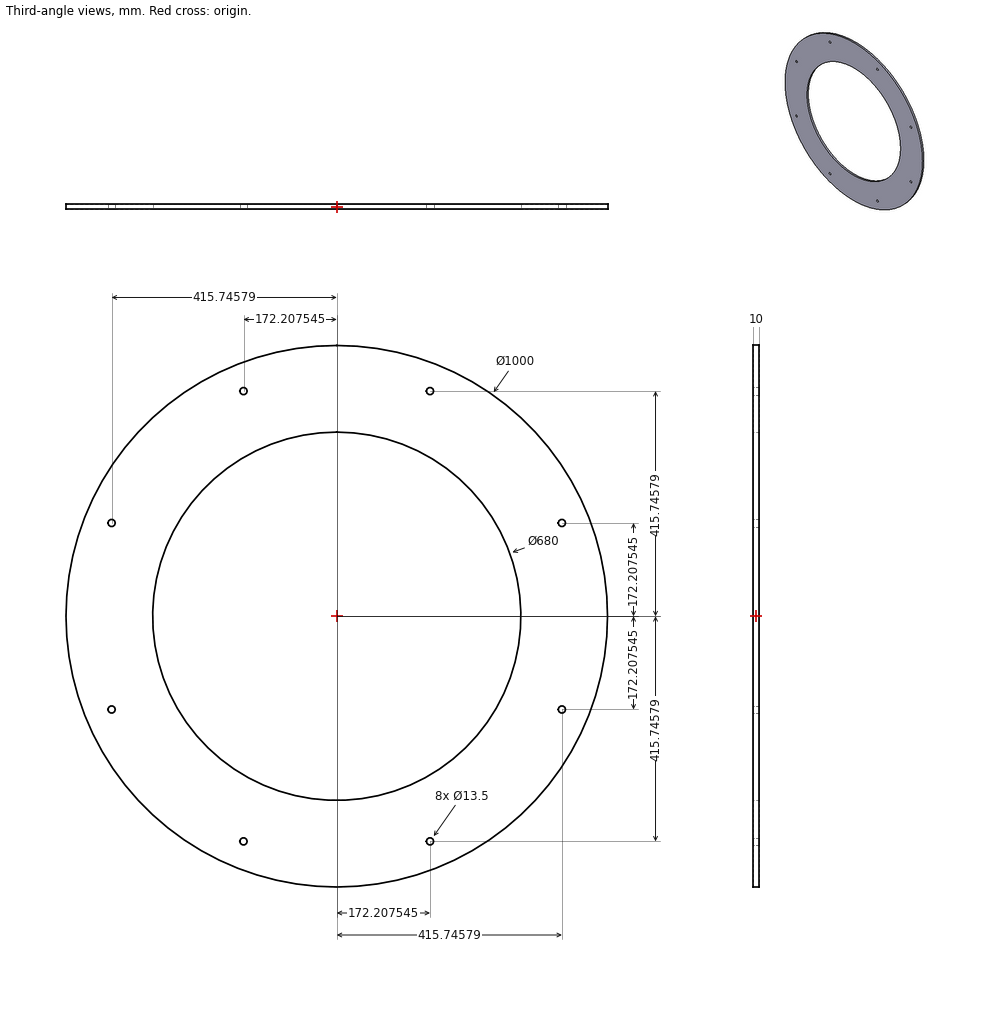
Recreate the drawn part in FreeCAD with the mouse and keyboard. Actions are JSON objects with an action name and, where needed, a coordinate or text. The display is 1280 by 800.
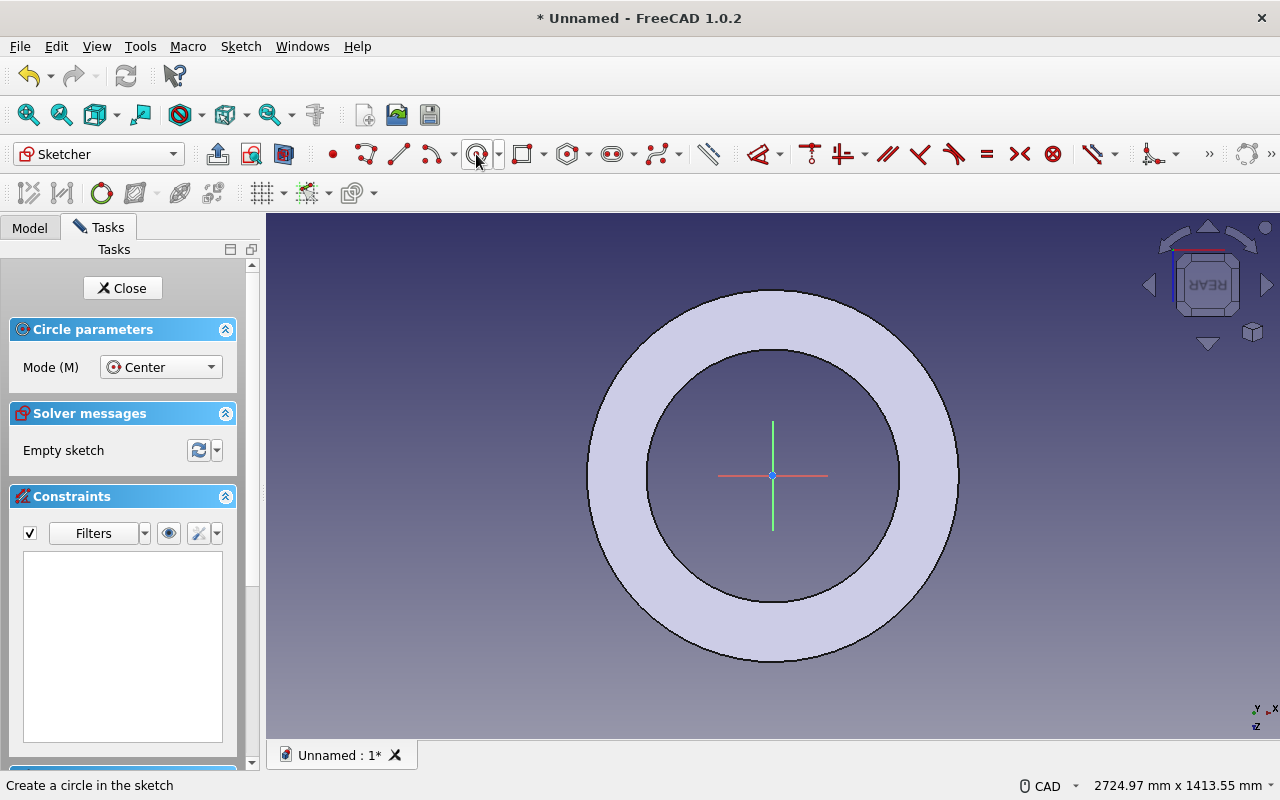
{"action": "scroll", "coordinate": [837, 321], "scroll_direction": "up", "scroll_amount": 12}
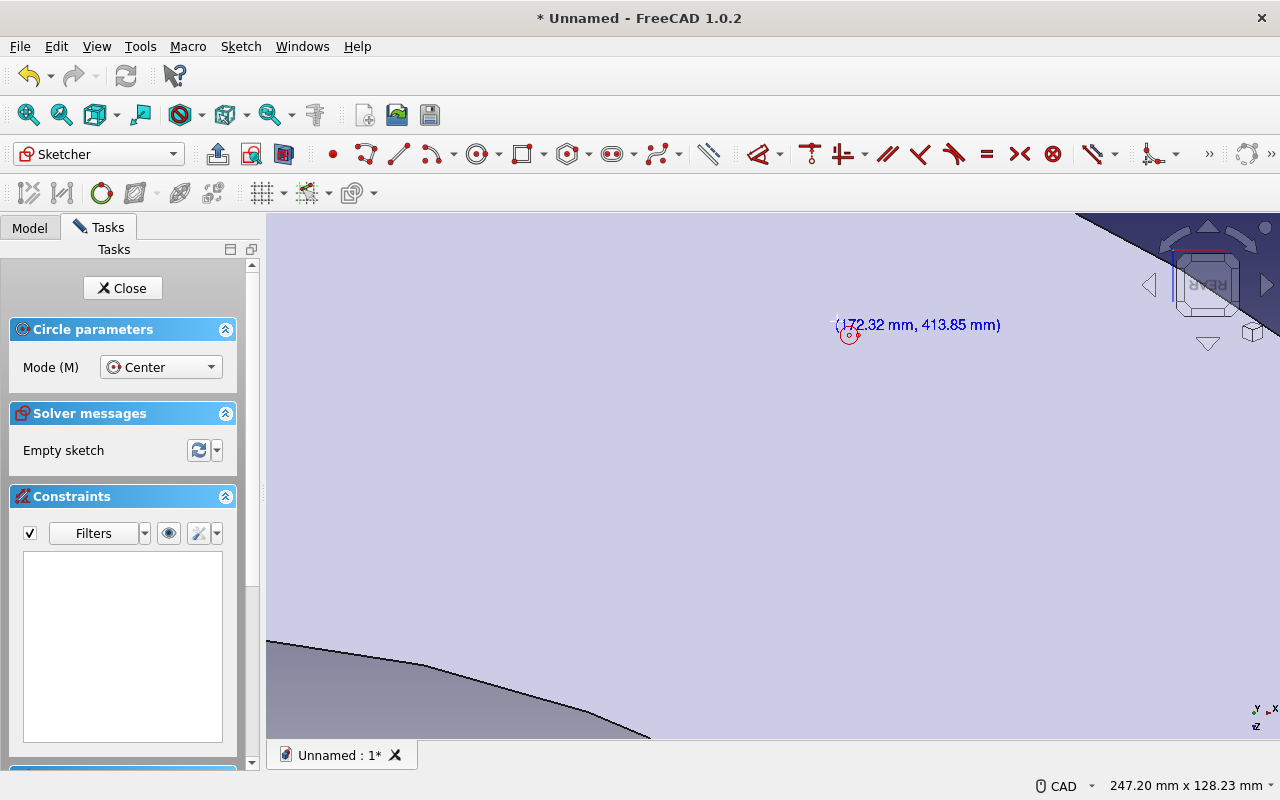
{"action": "scroll", "coordinate": [762, 321], "scroll_direction": "down", "scroll_amount": 12}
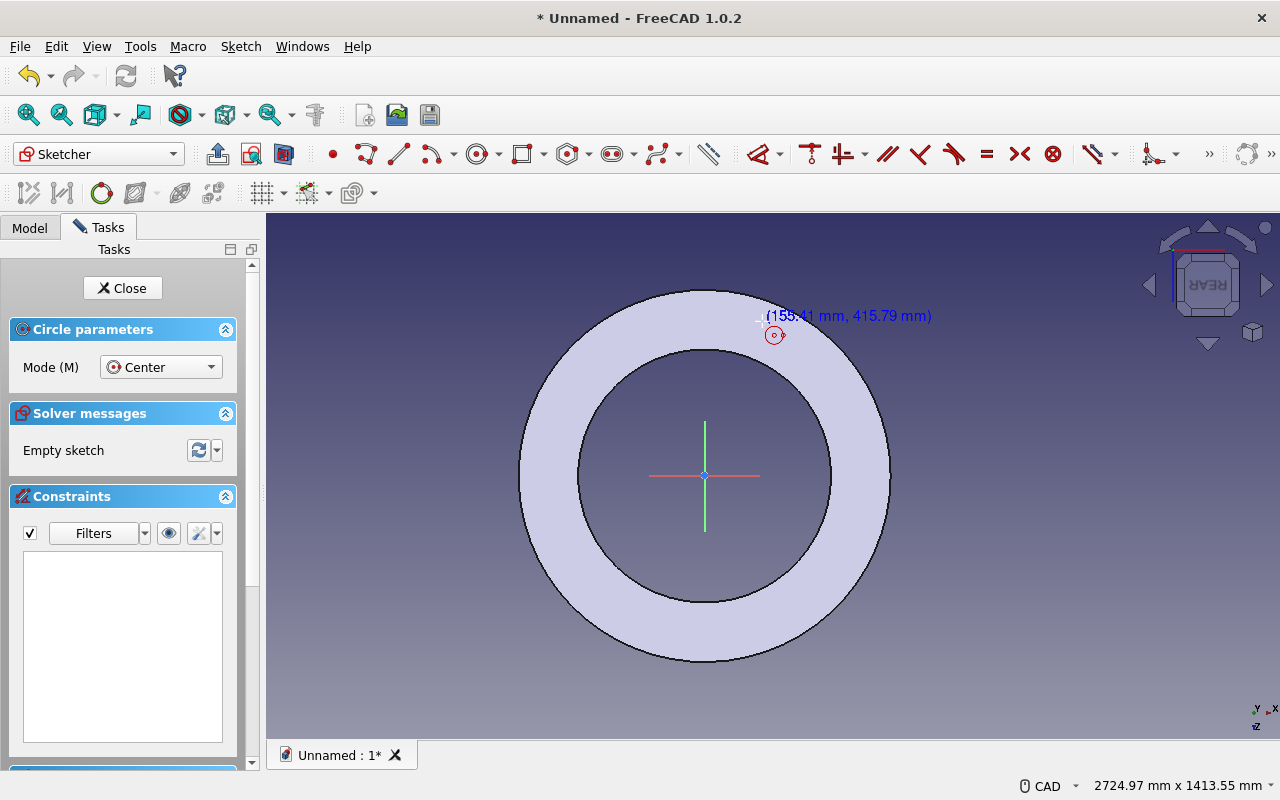
{"action": "left_click", "coordinate": [769, 321]}
{"action": "mouse_move", "coordinate": [770, 320]}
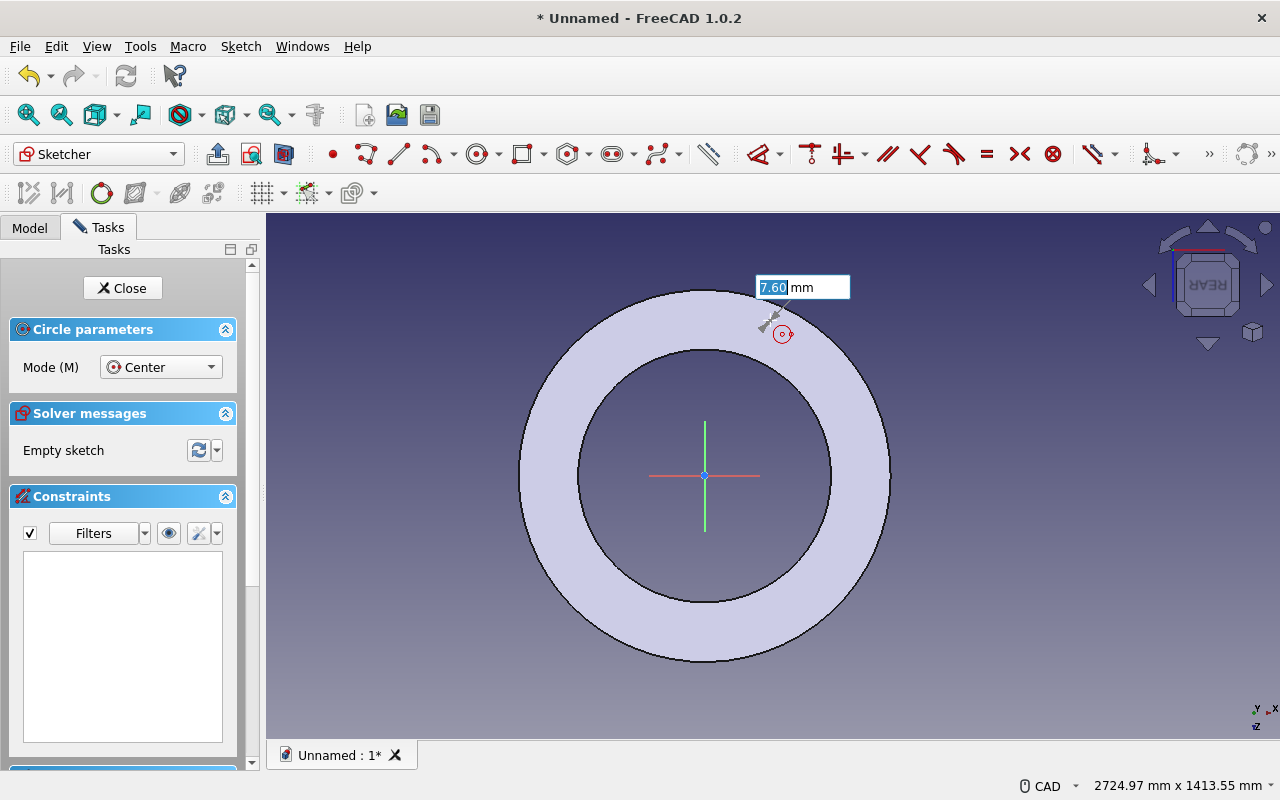
{"action": "type", "text": "13.5"}
{"action": "key", "text": "Return"}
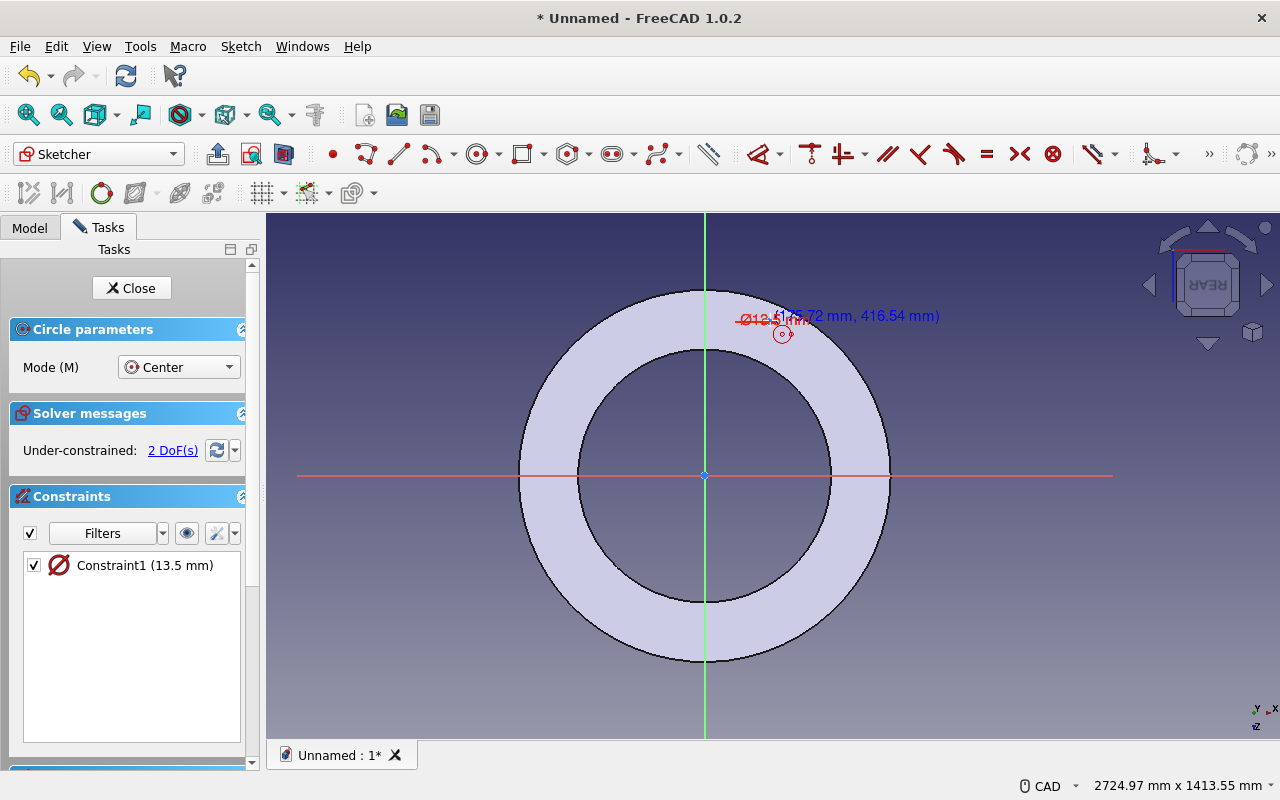
{"action": "scroll", "coordinate": [859, 412], "scroll_direction": "up", "scroll_amount": 12}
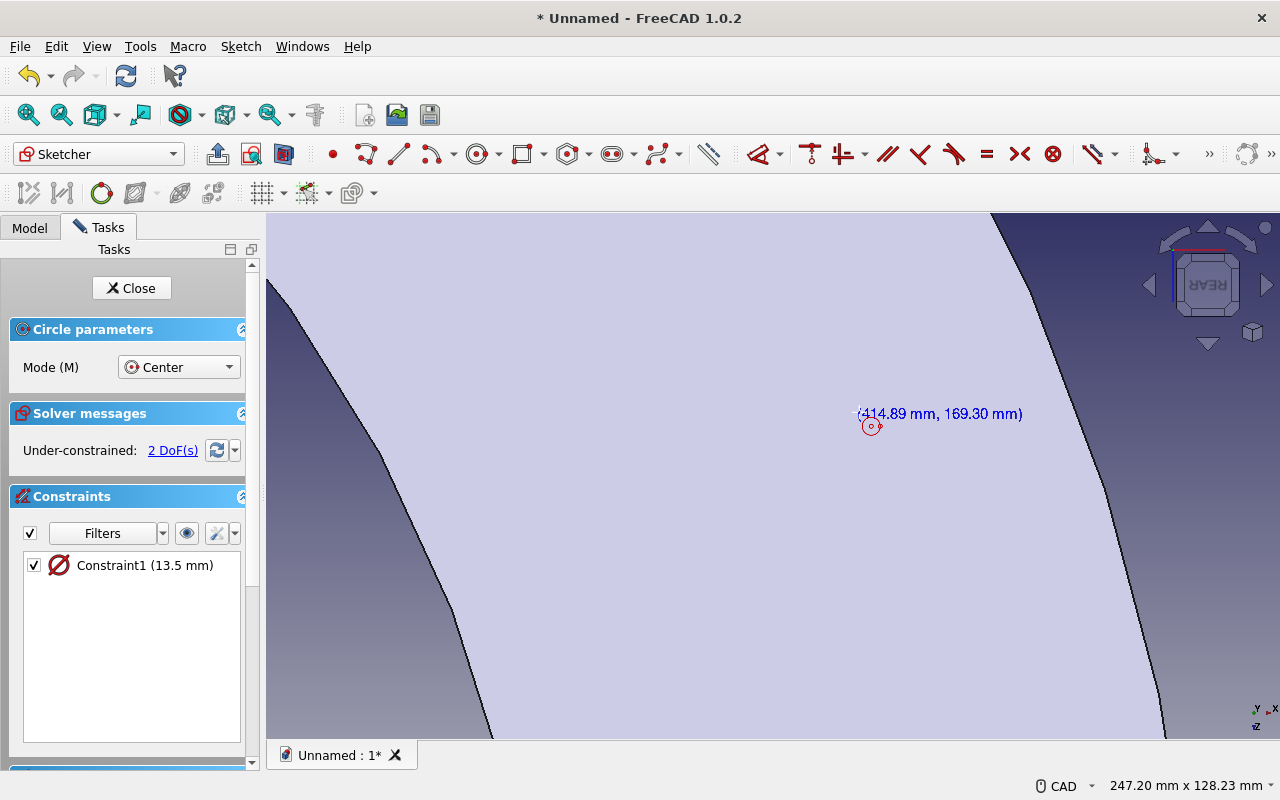
{"action": "scroll", "coordinate": [859, 412], "scroll_direction": "down", "scroll_amount": 12}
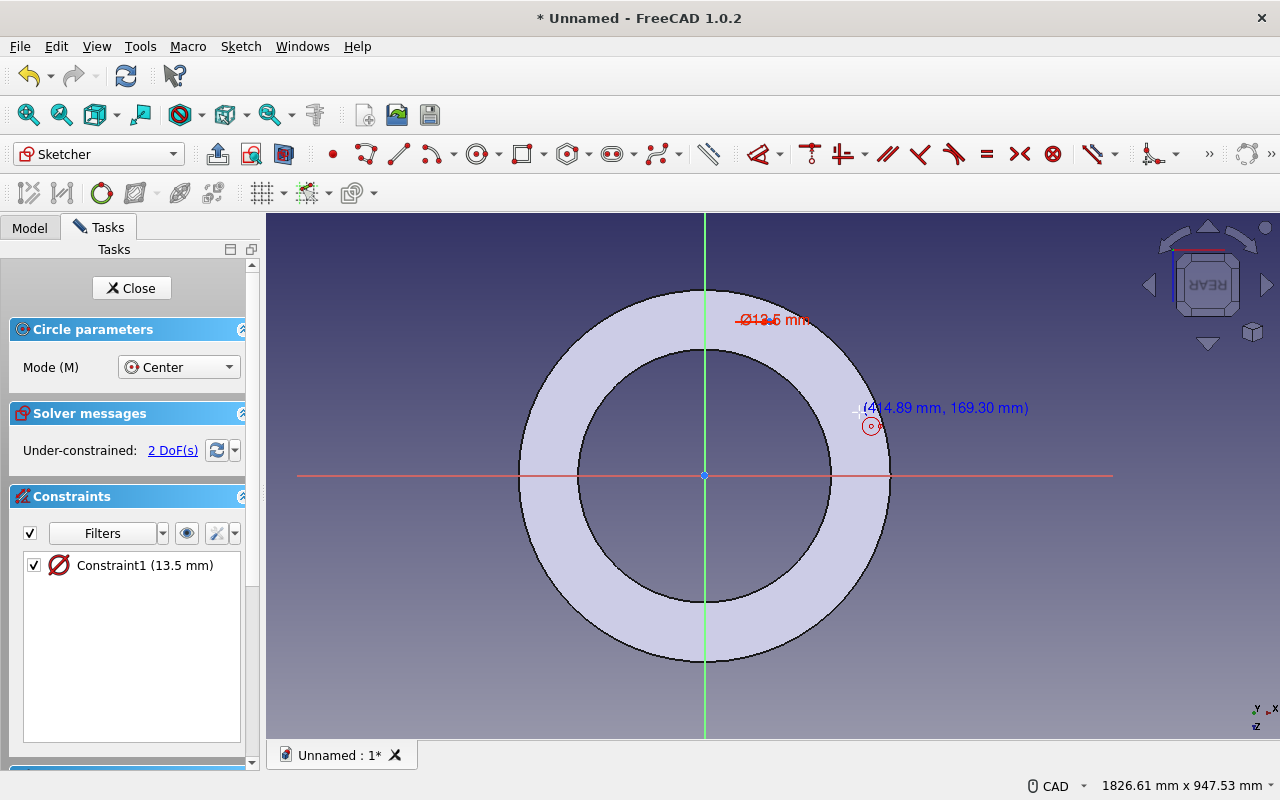
{"action": "left_click", "coordinate": [859, 412]}
{"action": "mouse_move", "coordinate": [861, 410]}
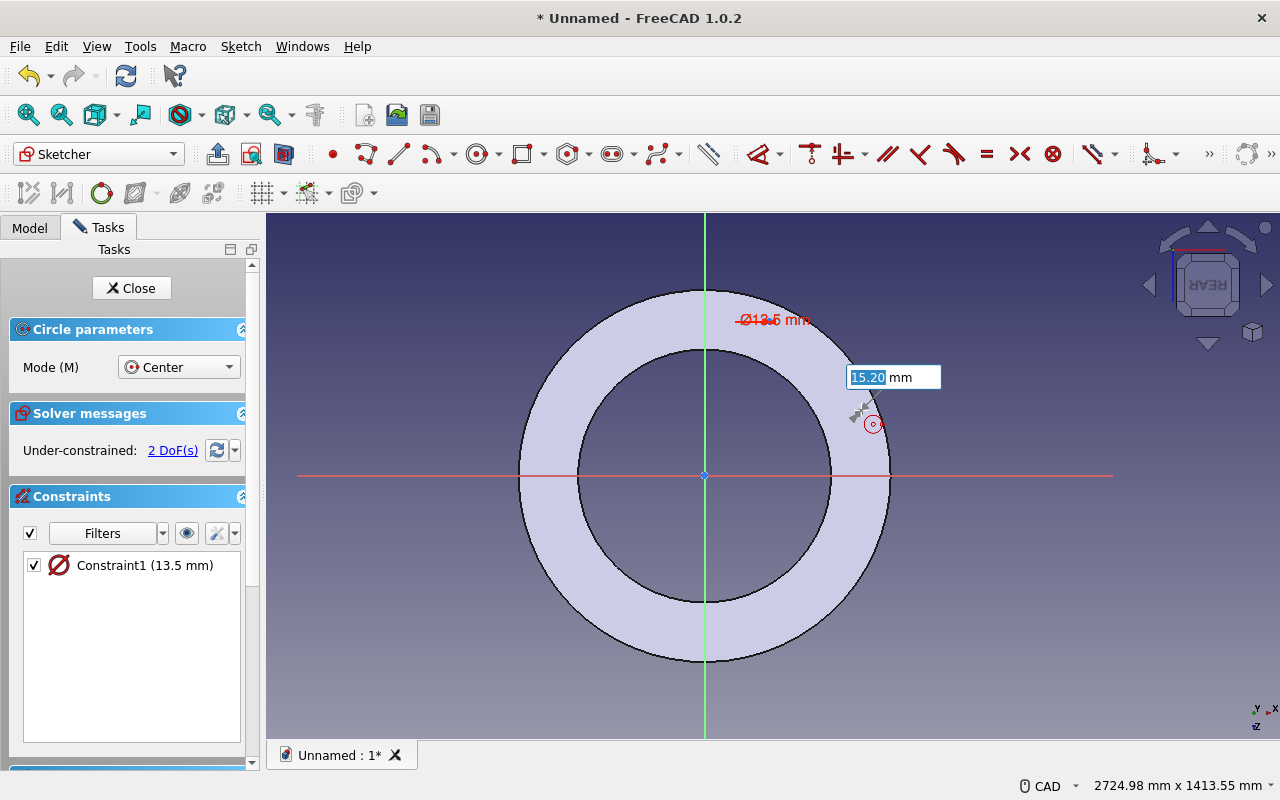
{"action": "type", "text": "13.5"}
{"action": "key", "text": "Return"}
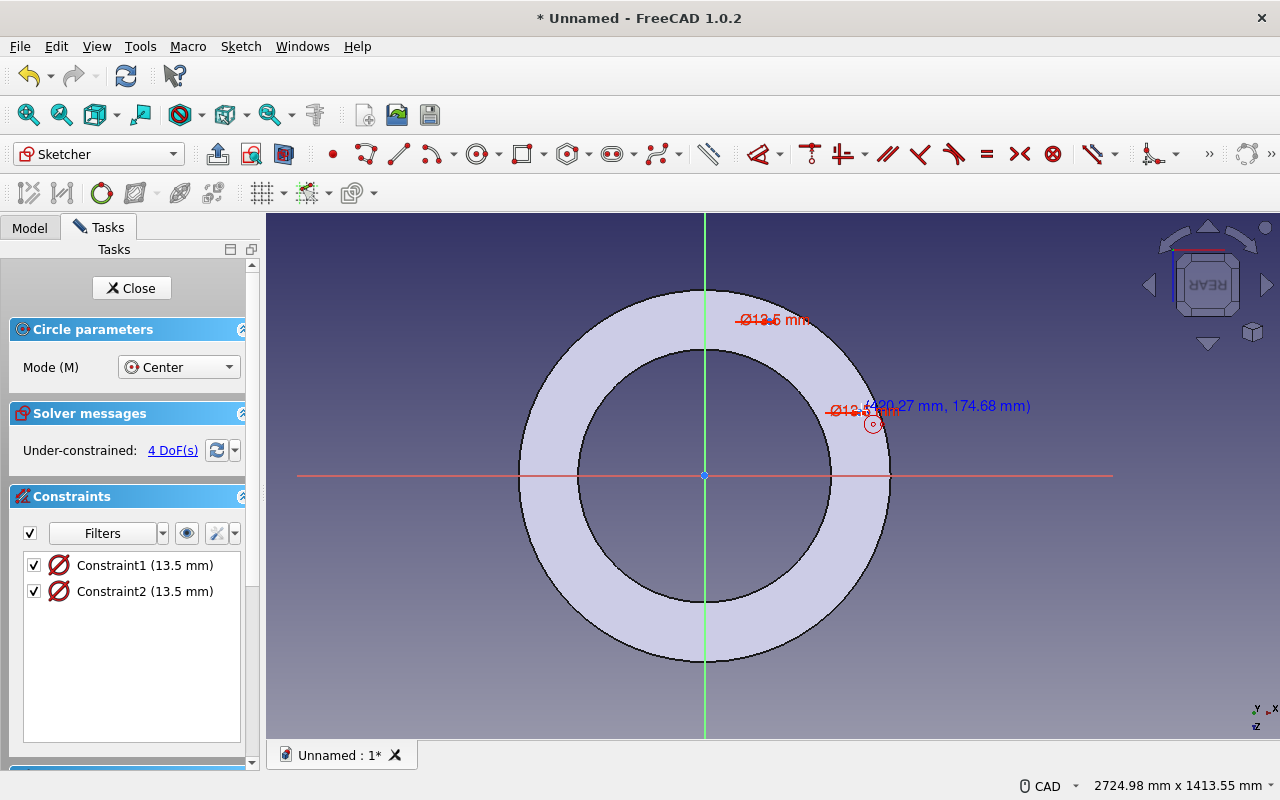
{"action": "scroll", "coordinate": [859, 540], "scroll_direction": "up", "scroll_amount": 12}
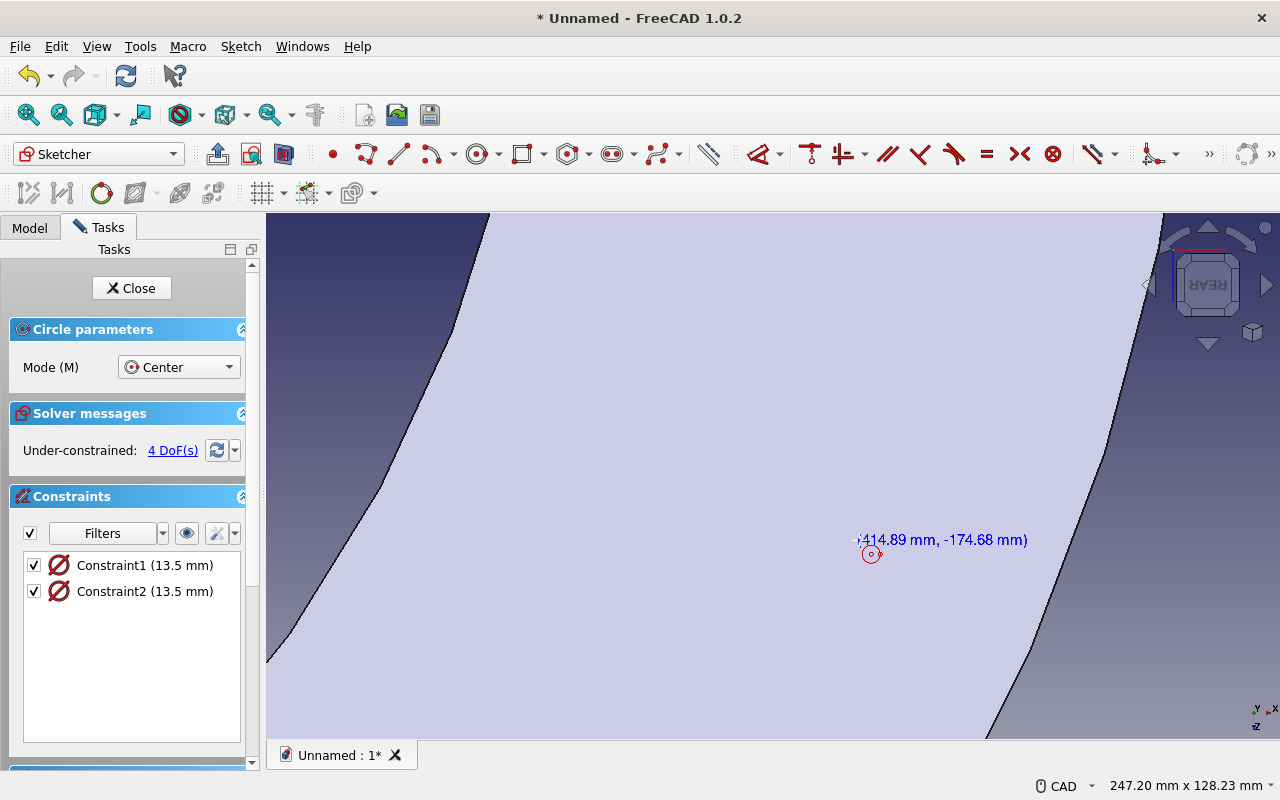
{"action": "scroll", "coordinate": [859, 541], "scroll_direction": "down", "scroll_amount": 12}